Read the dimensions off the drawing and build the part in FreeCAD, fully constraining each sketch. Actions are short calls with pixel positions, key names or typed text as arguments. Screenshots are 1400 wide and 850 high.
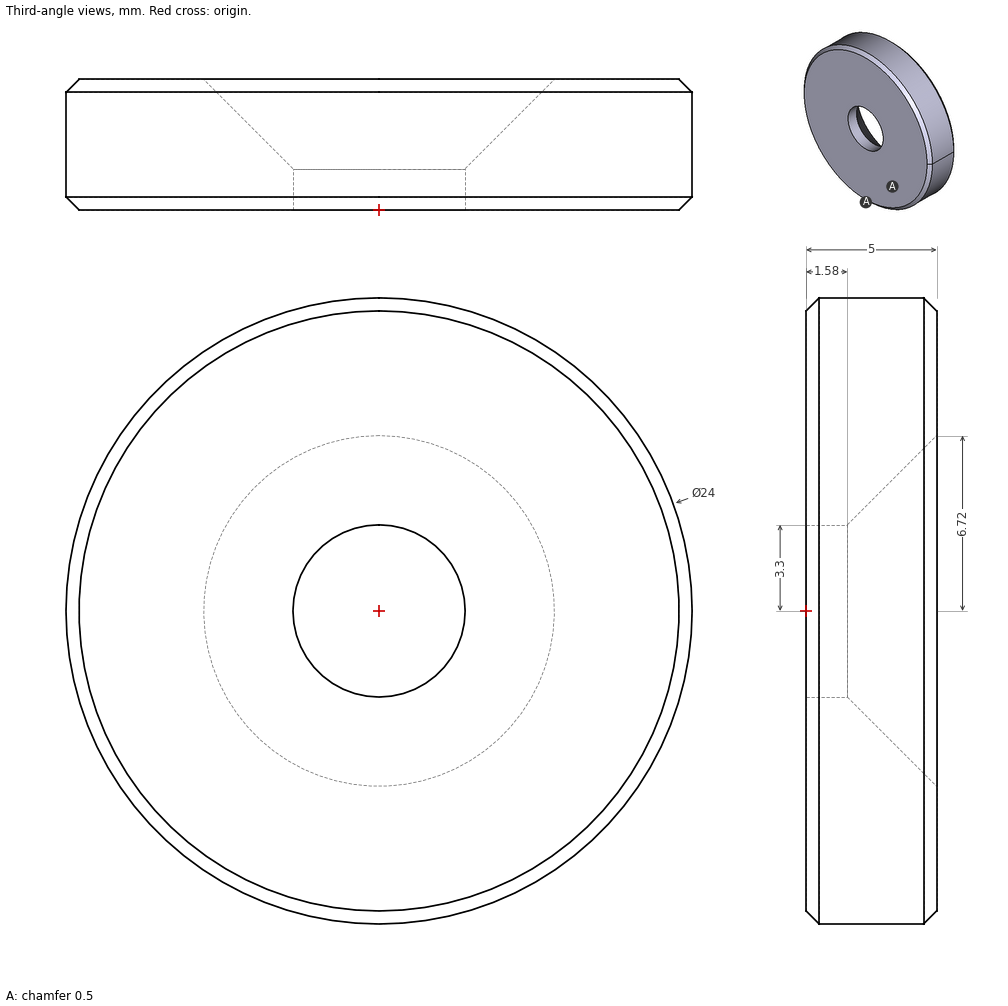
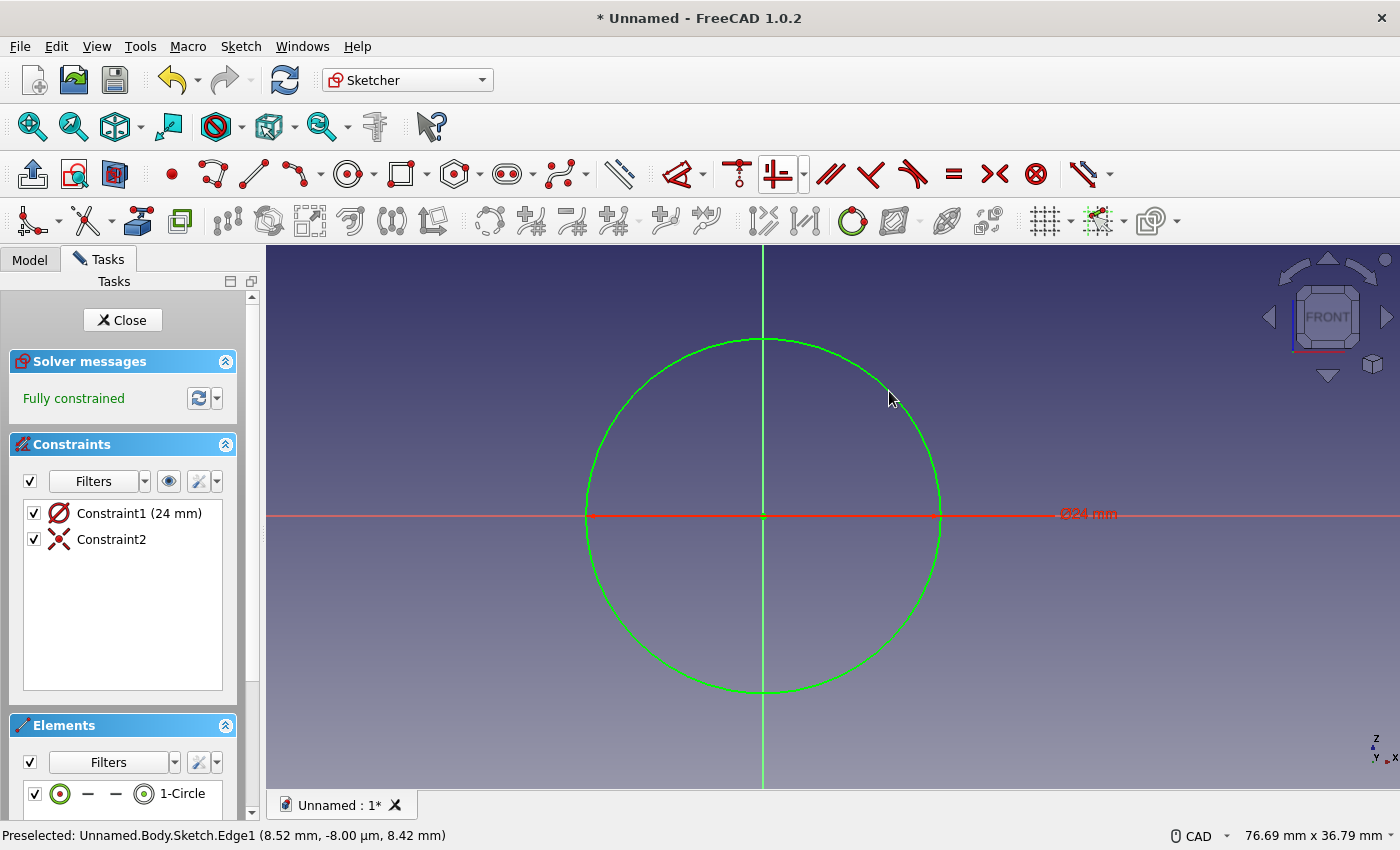
click(123, 320)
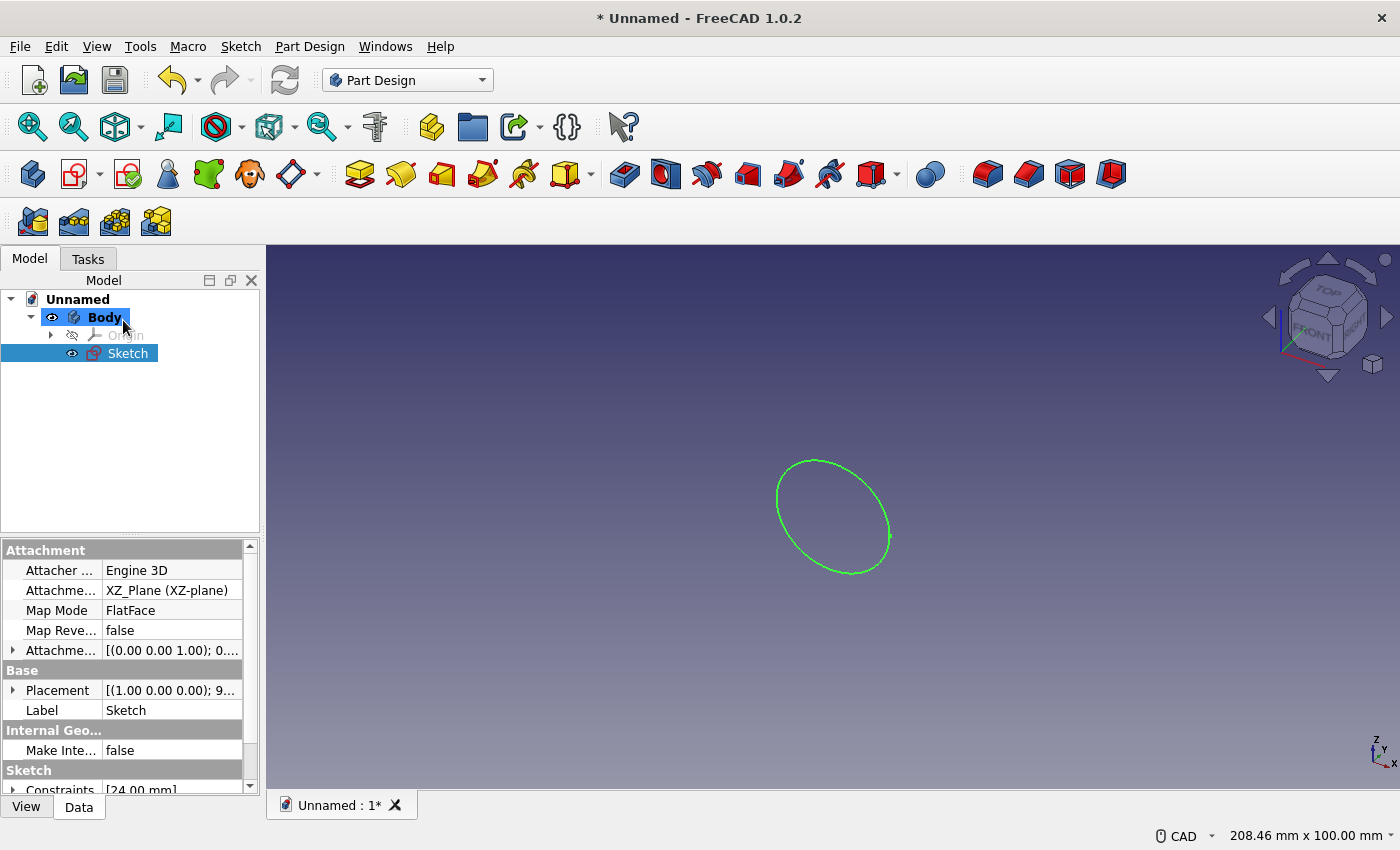
click(360, 174)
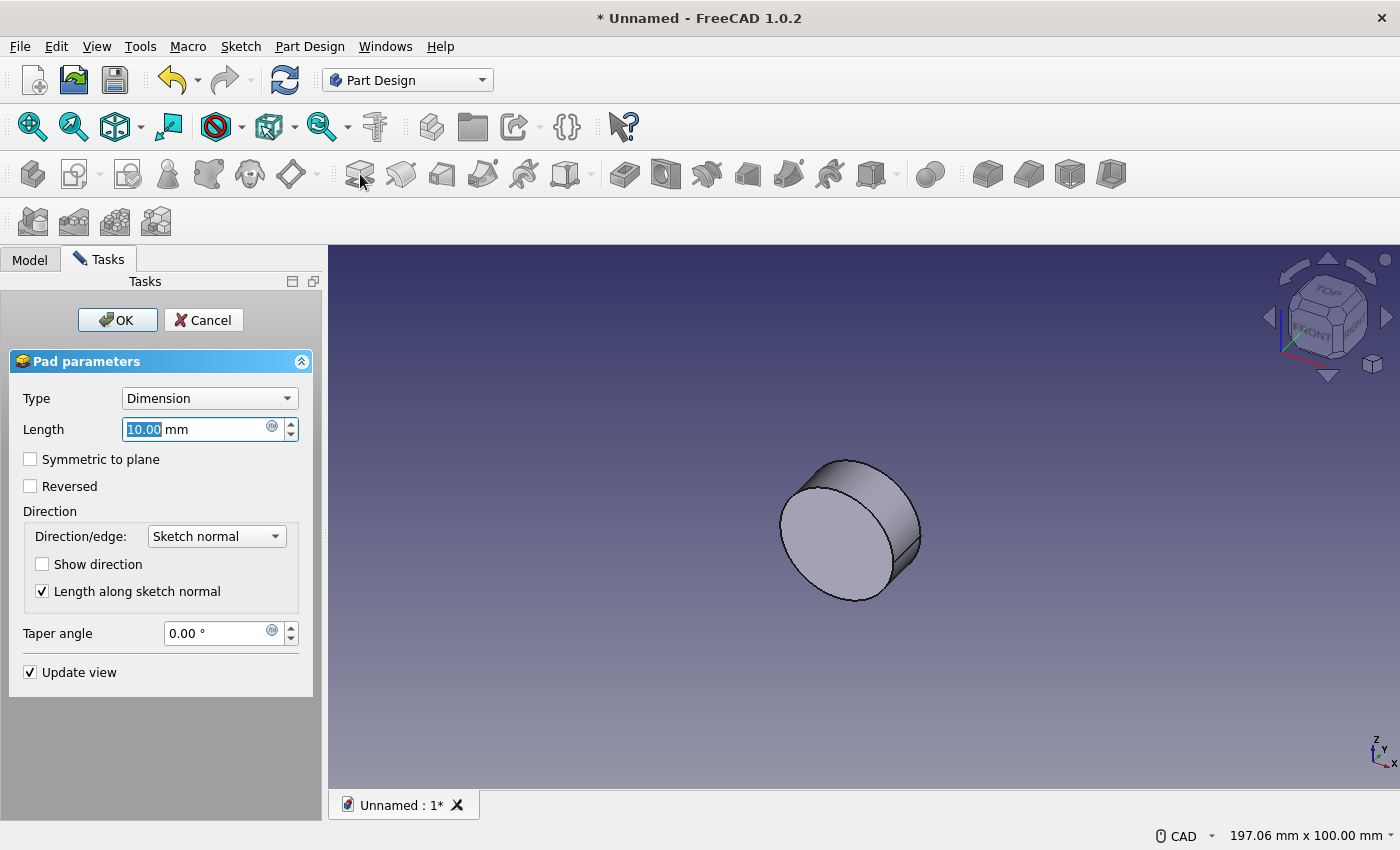
text(5)
key(Tab)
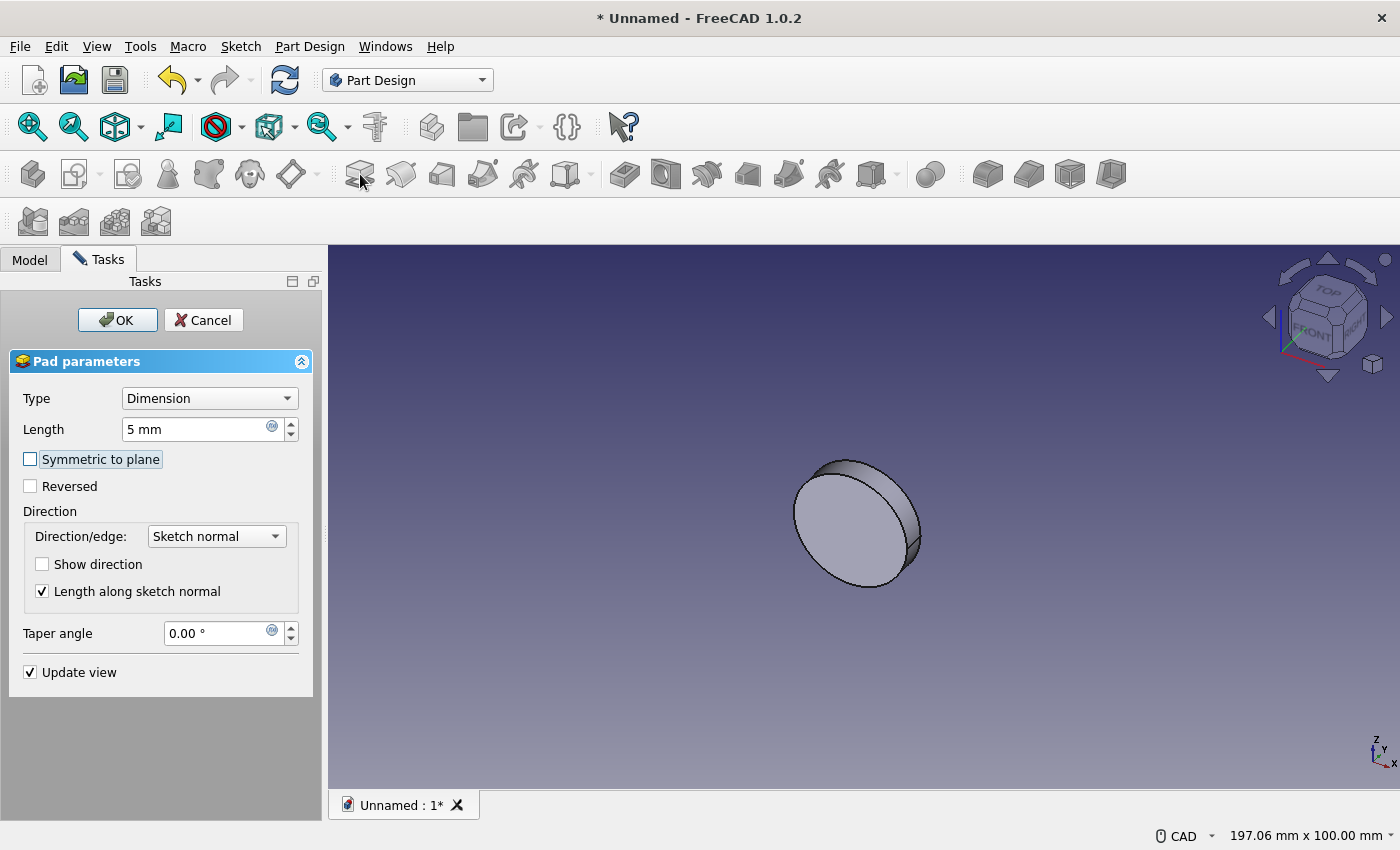
click(31, 486)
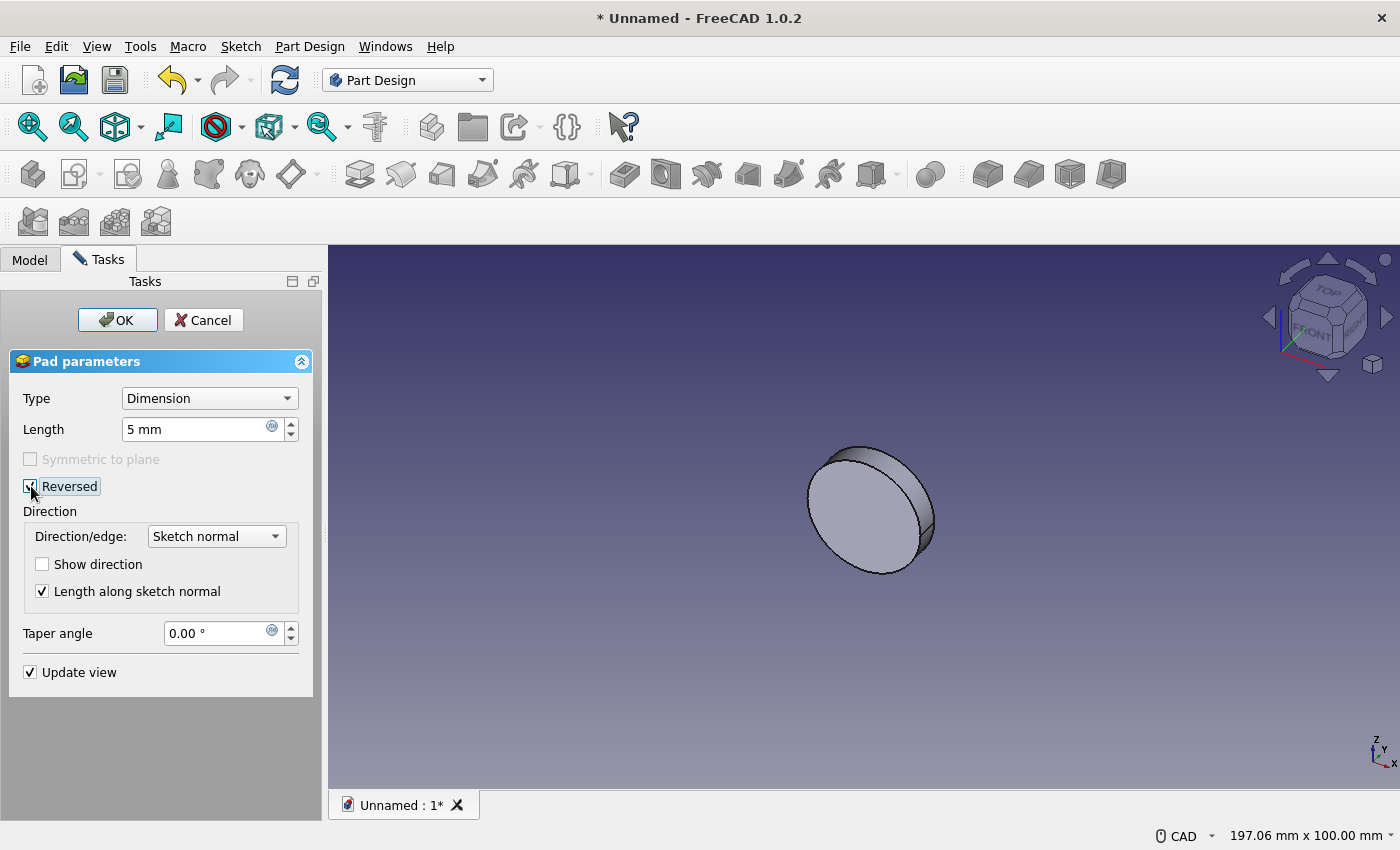
click(118, 320)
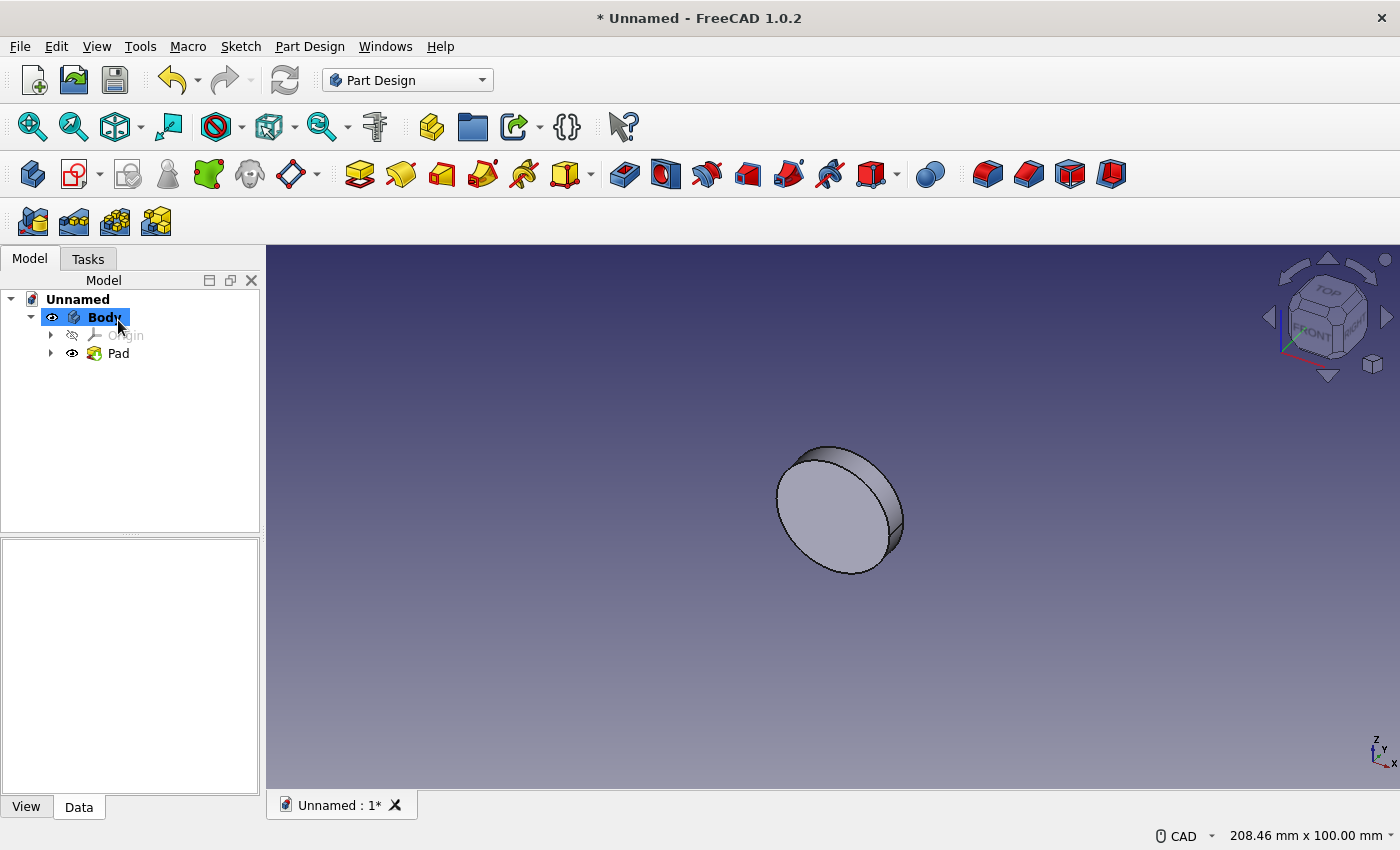
click(33, 128)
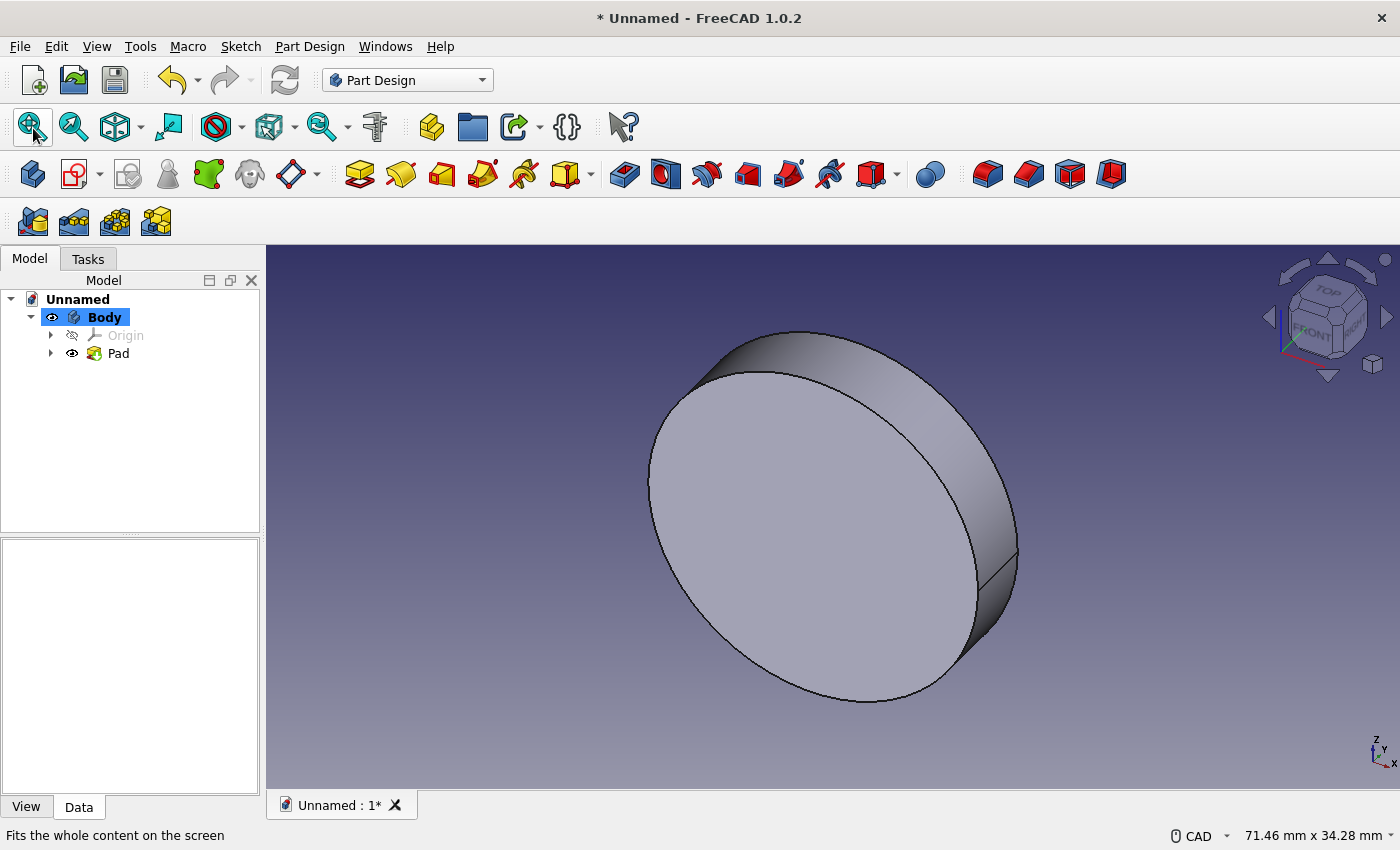
click(74, 174)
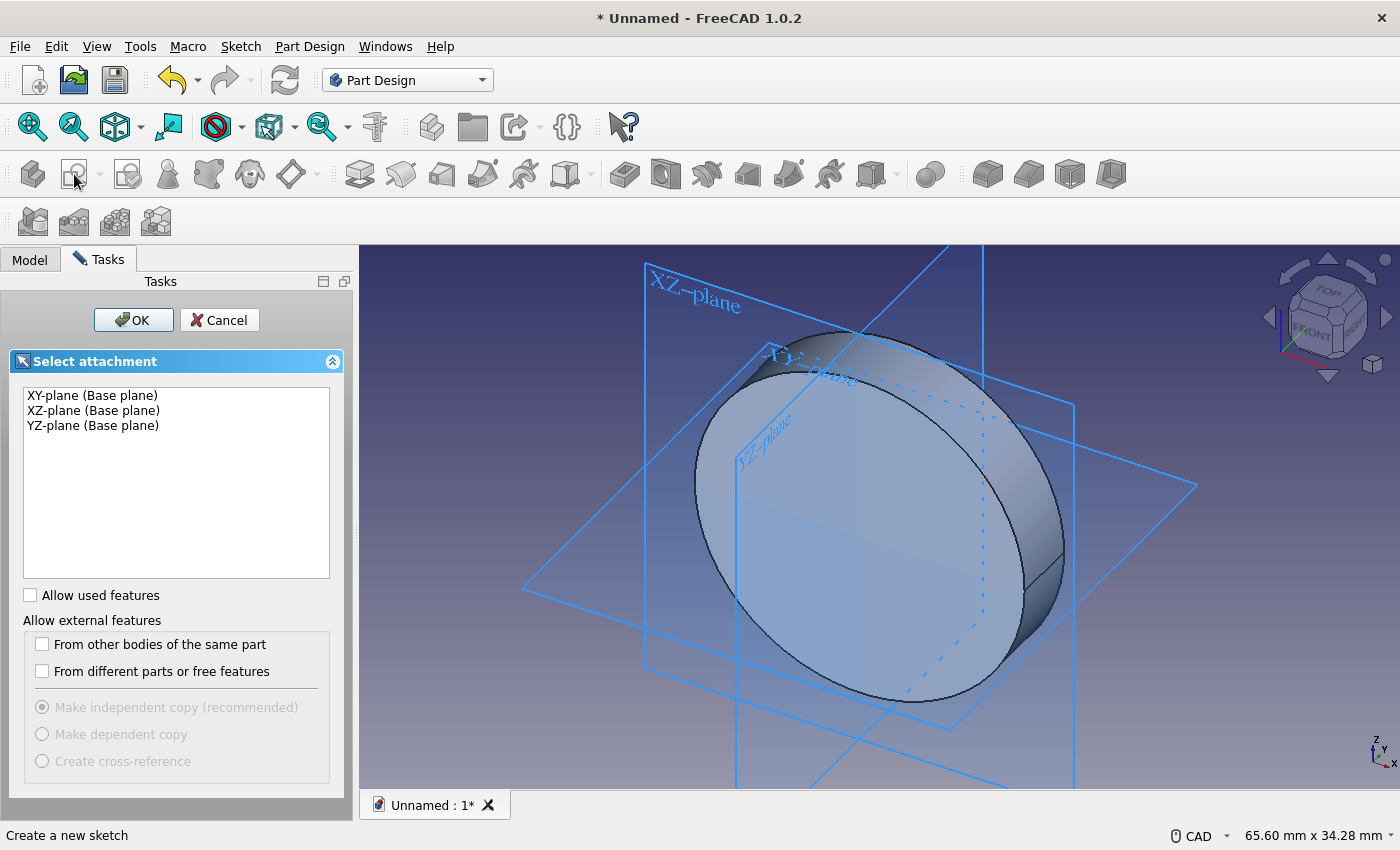
click(84, 426)